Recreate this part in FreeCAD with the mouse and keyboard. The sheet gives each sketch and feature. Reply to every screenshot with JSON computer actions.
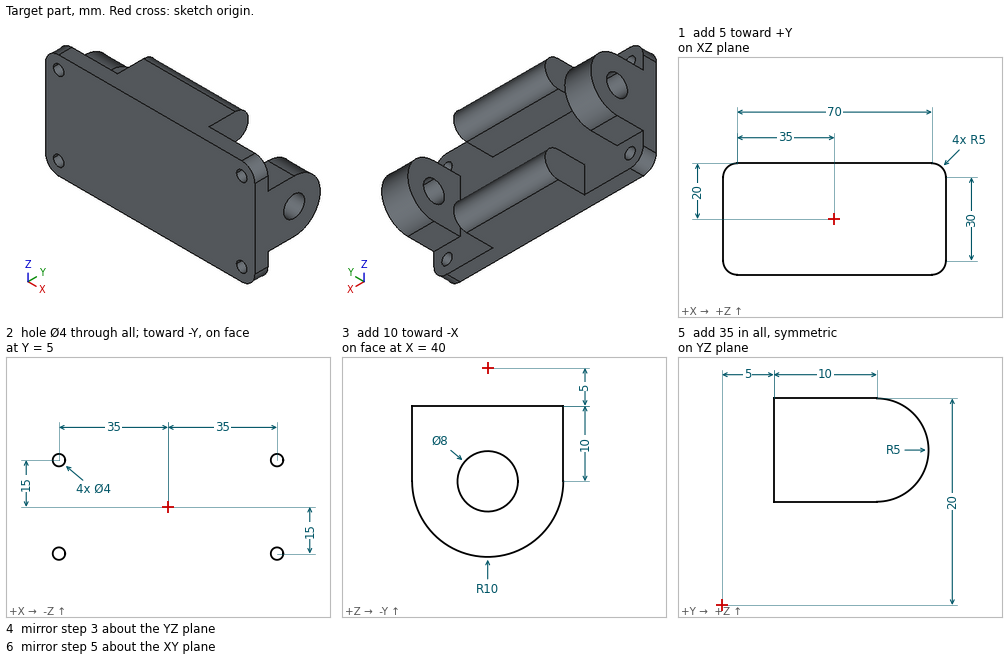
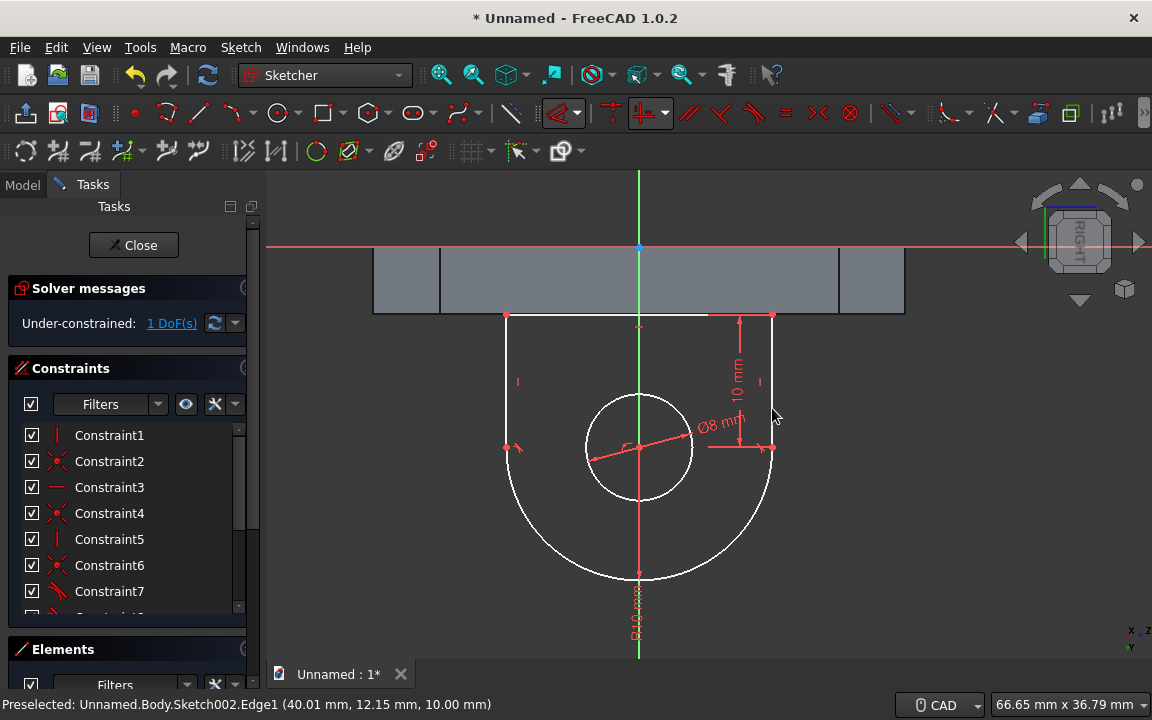
{"action": "left_click", "coordinate": [772, 315]}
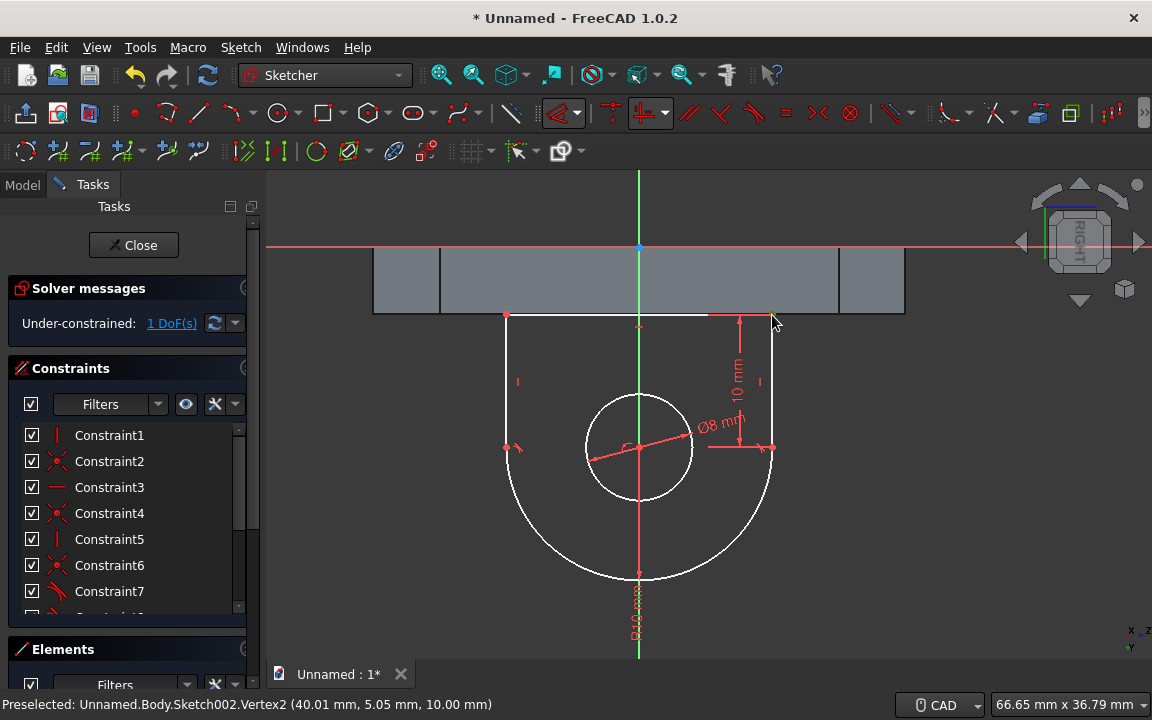
{"action": "left_click", "coordinate": [580, 114]}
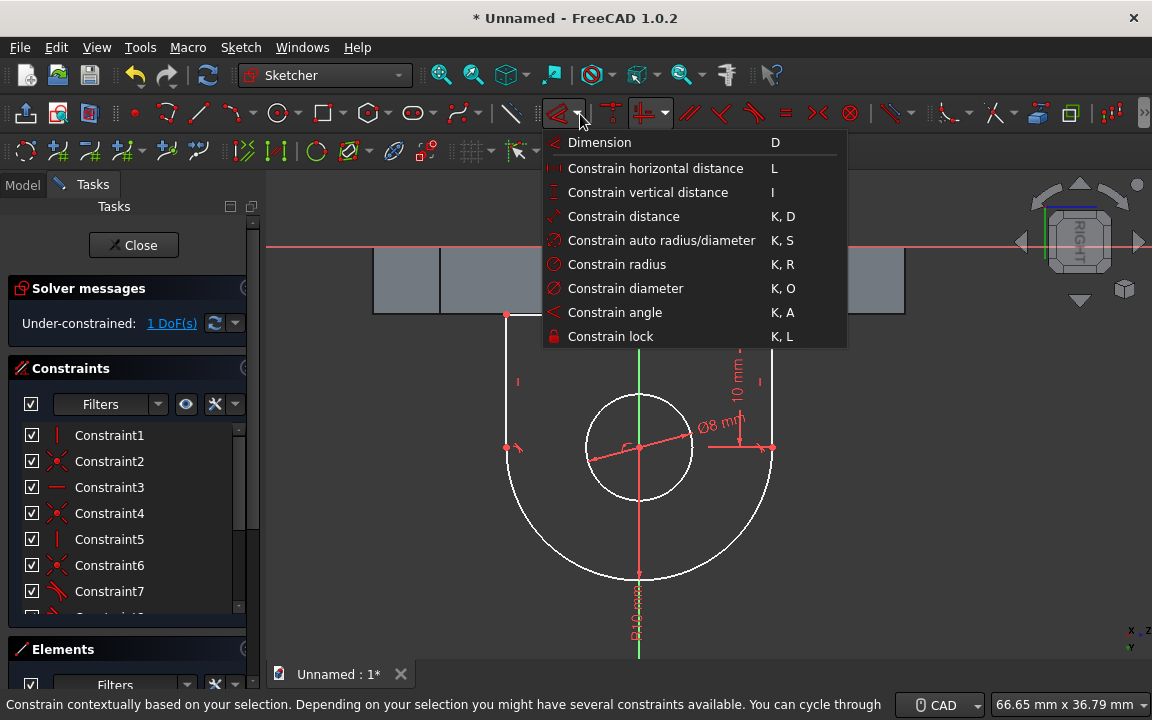
{"action": "left_click", "coordinate": [695, 192]}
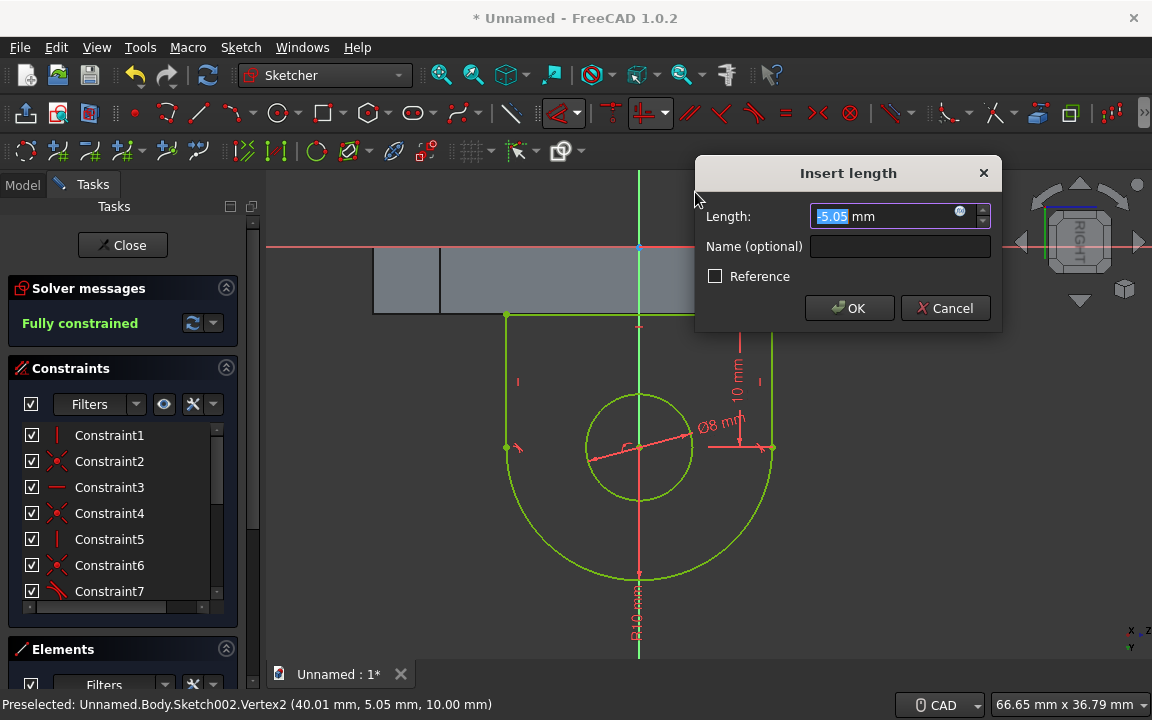
{"action": "type", "text": "-5"}
{"action": "key", "text": "Return"}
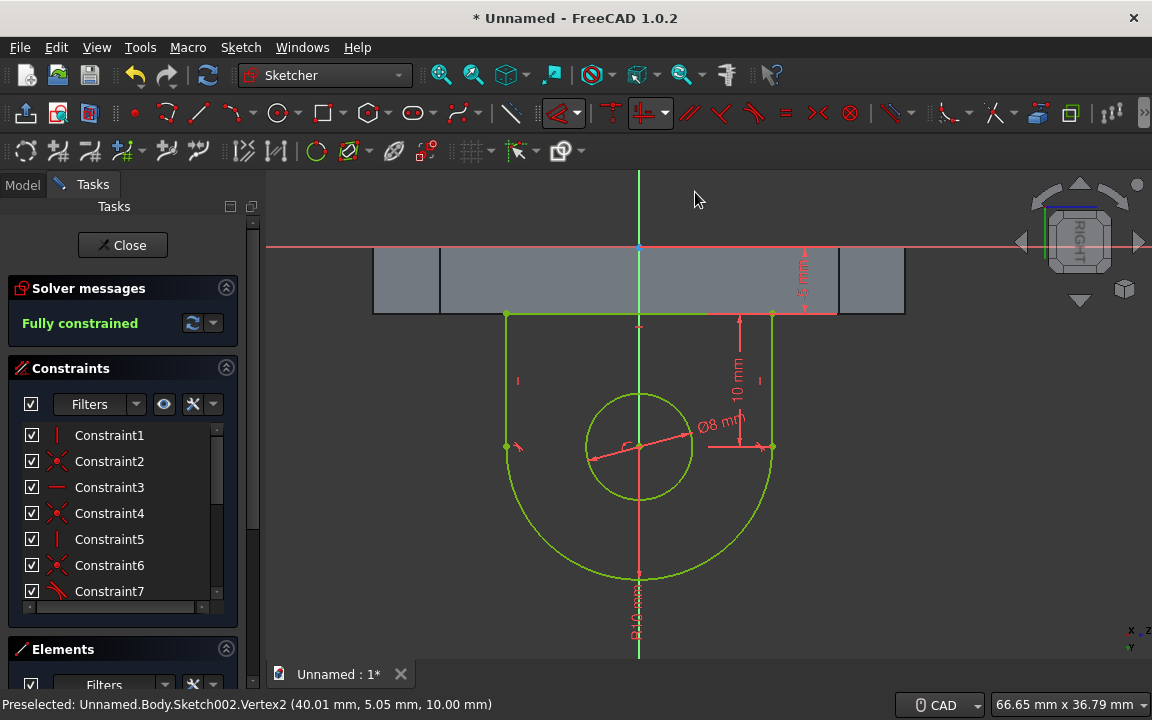
{"action": "left_click", "coordinate": [123, 245]}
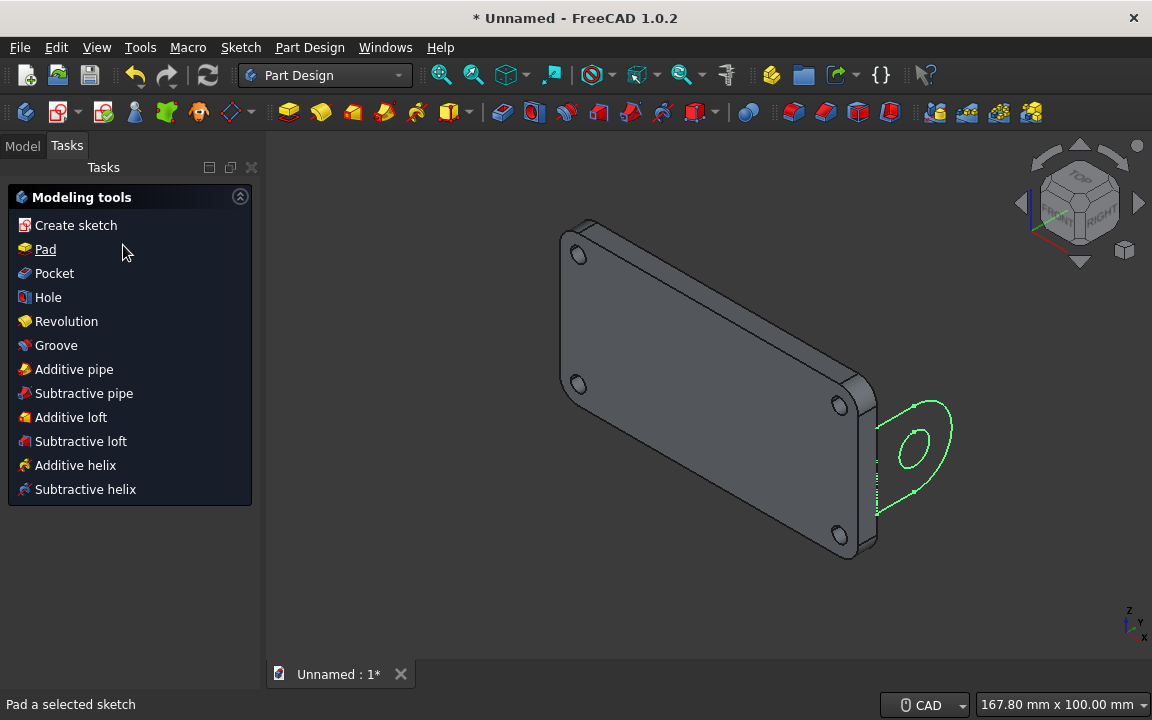
{"action": "left_click", "coordinate": [290, 112]}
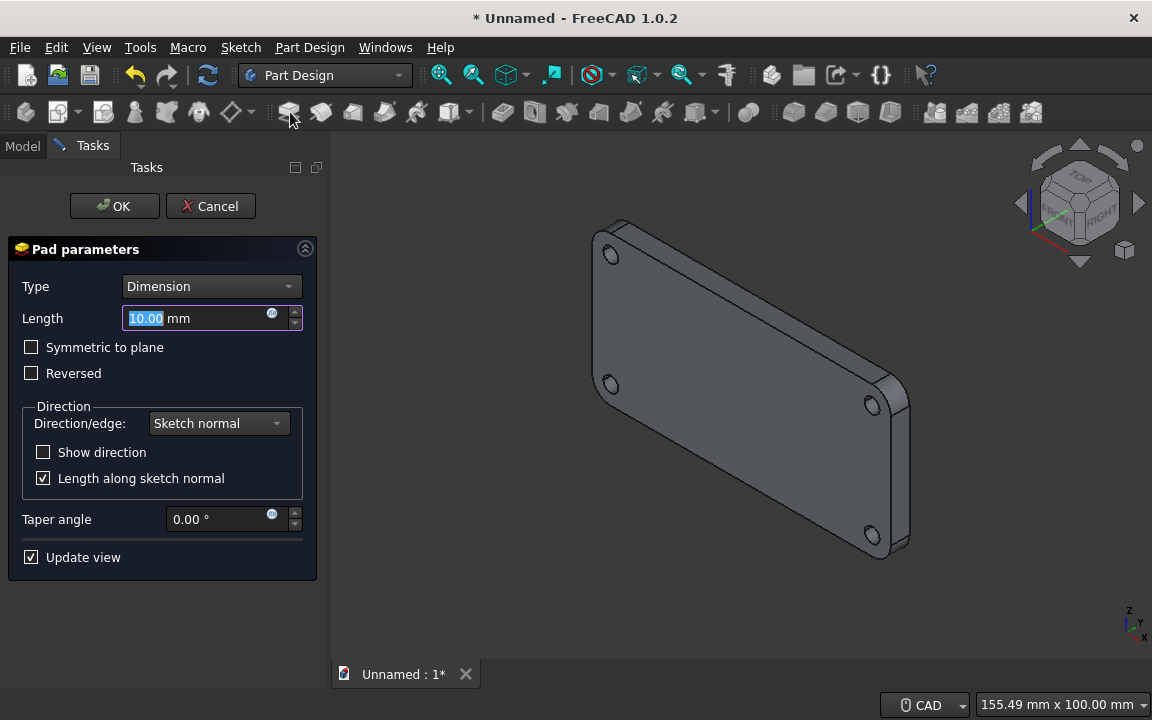
{"action": "type", "text": "10"}
{"action": "key", "text": "Tab"}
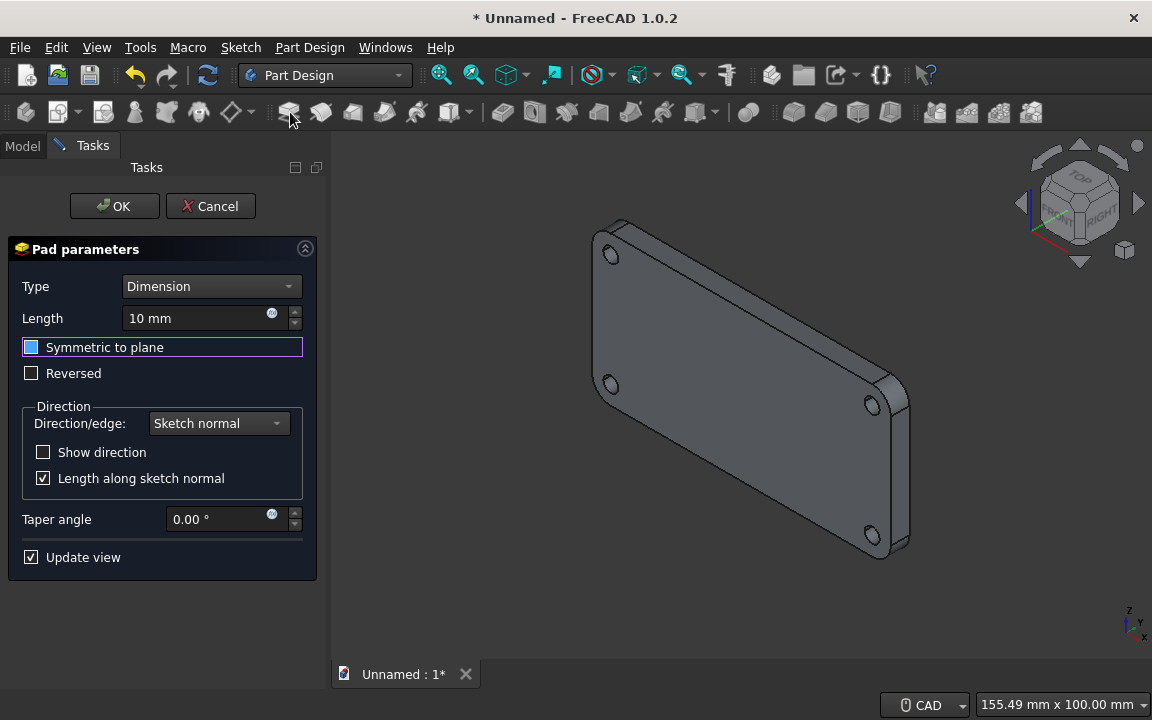
{"action": "left_click", "coordinate": [30, 373]}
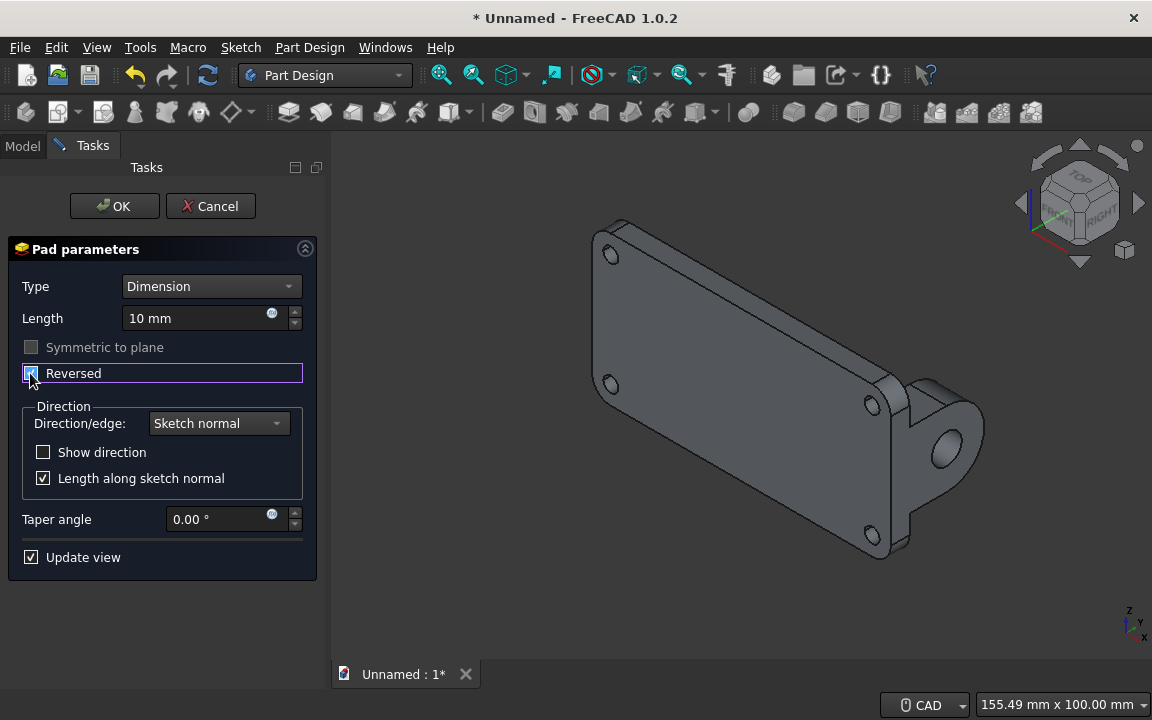
{"action": "left_click", "coordinate": [115, 206]}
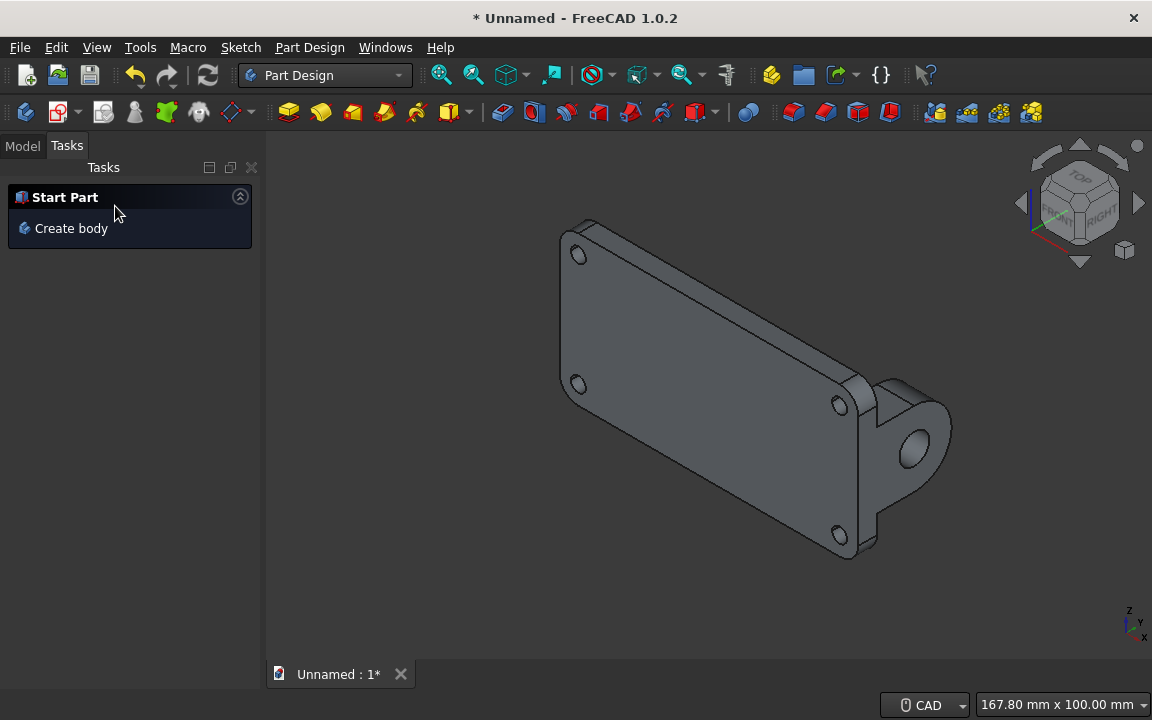
{"action": "left_click", "coordinate": [23, 145]}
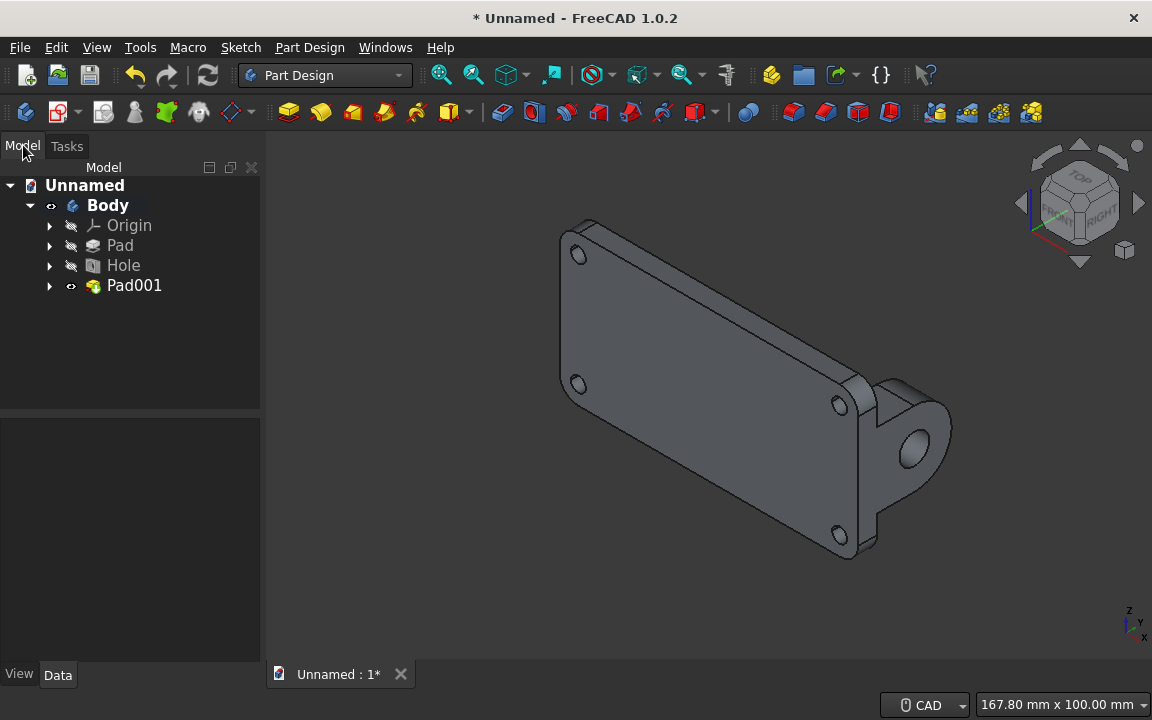
{"action": "left_click", "coordinate": [116, 286]}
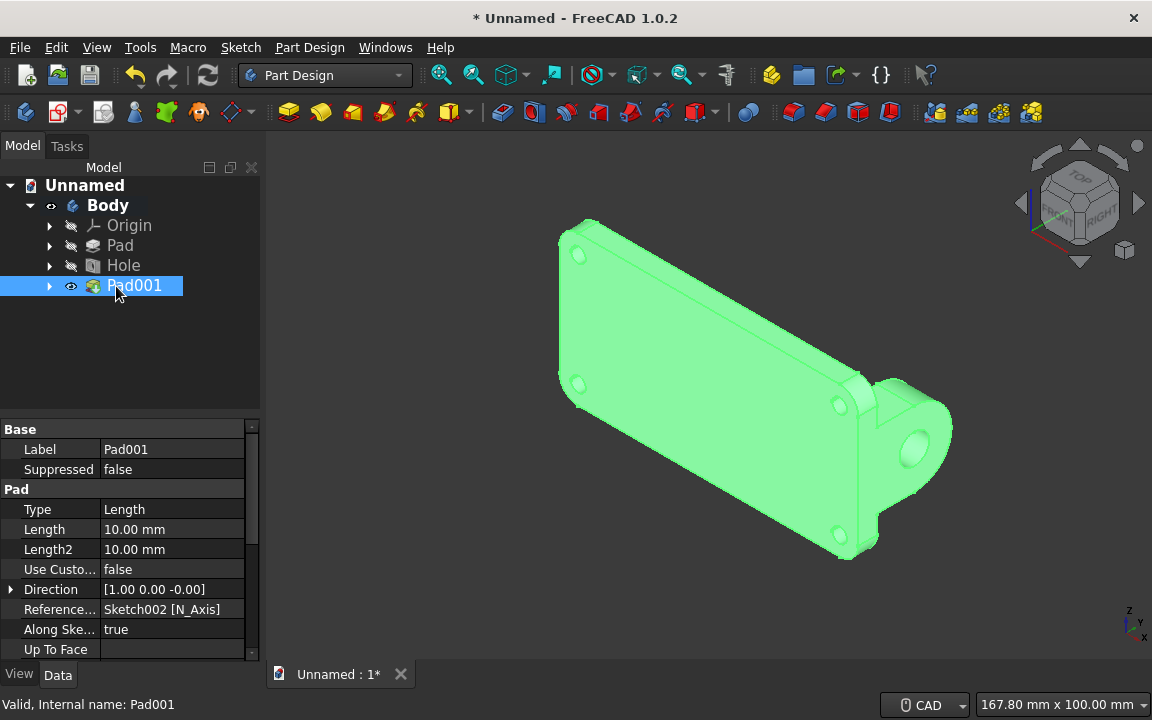
{"action": "left_click", "coordinate": [936, 112]}